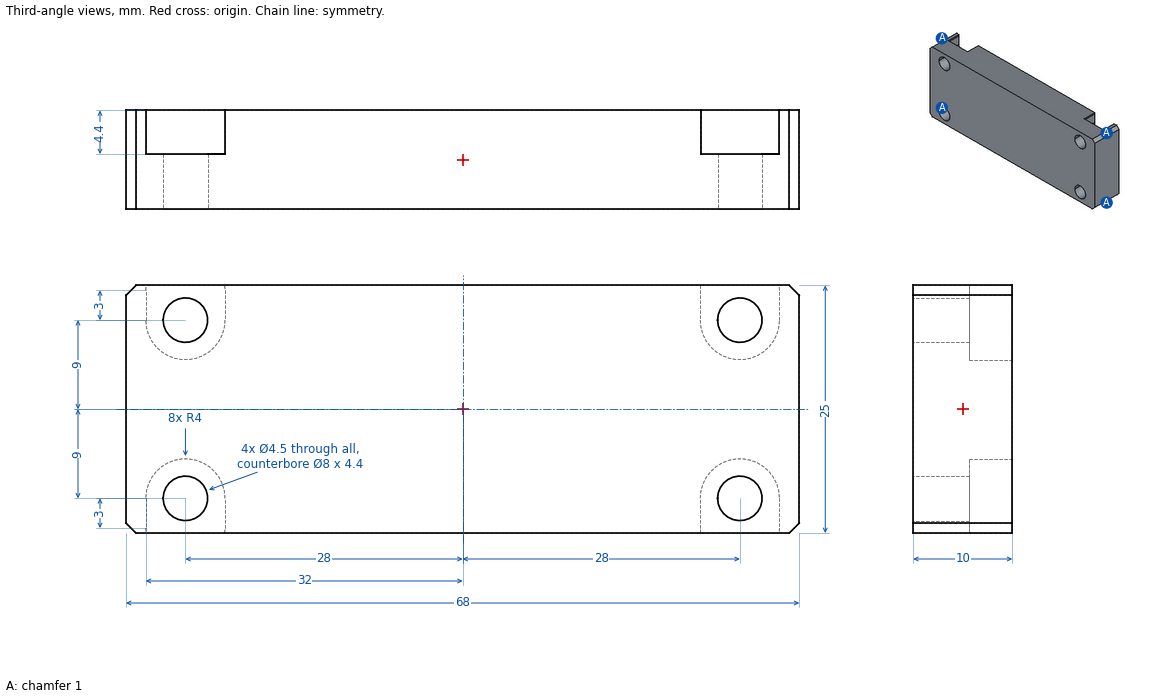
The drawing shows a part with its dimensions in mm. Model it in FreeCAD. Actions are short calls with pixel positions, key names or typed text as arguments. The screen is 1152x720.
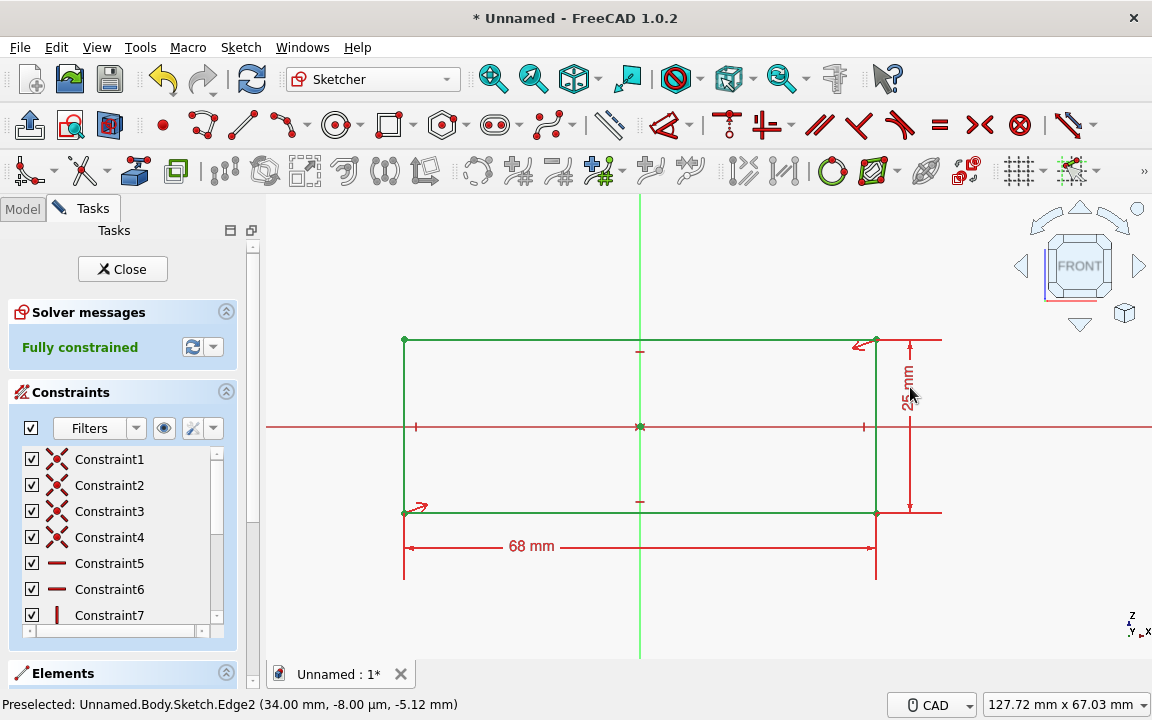
click(123, 269)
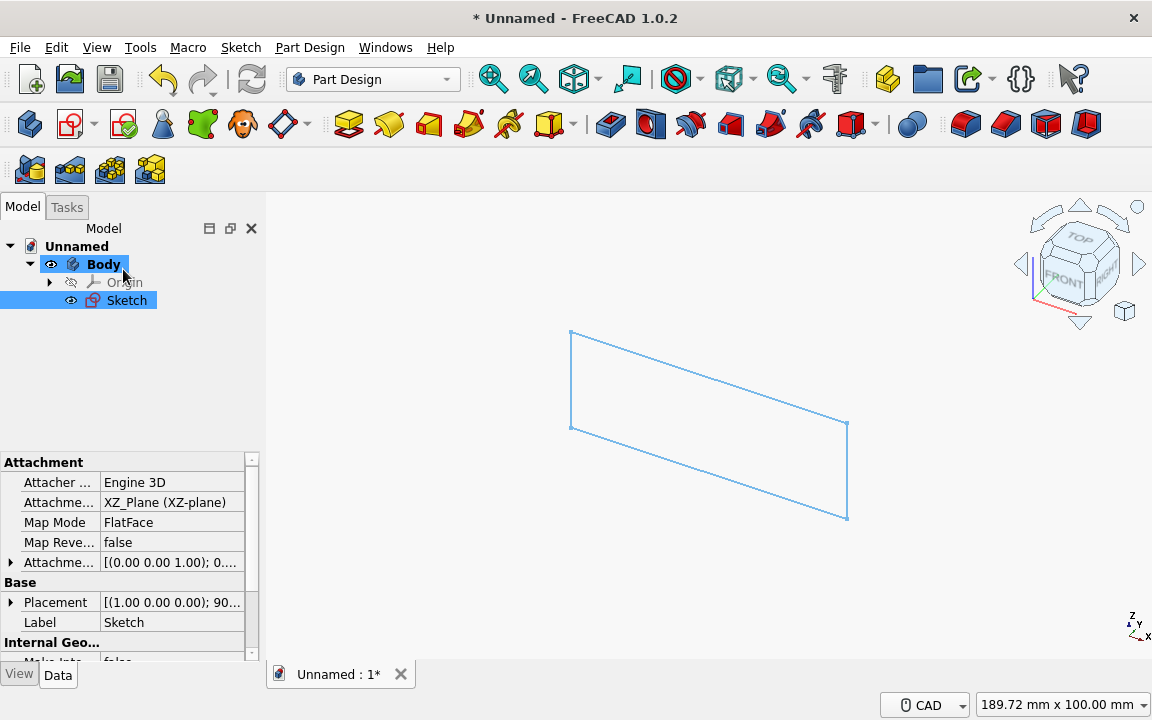
click(350, 124)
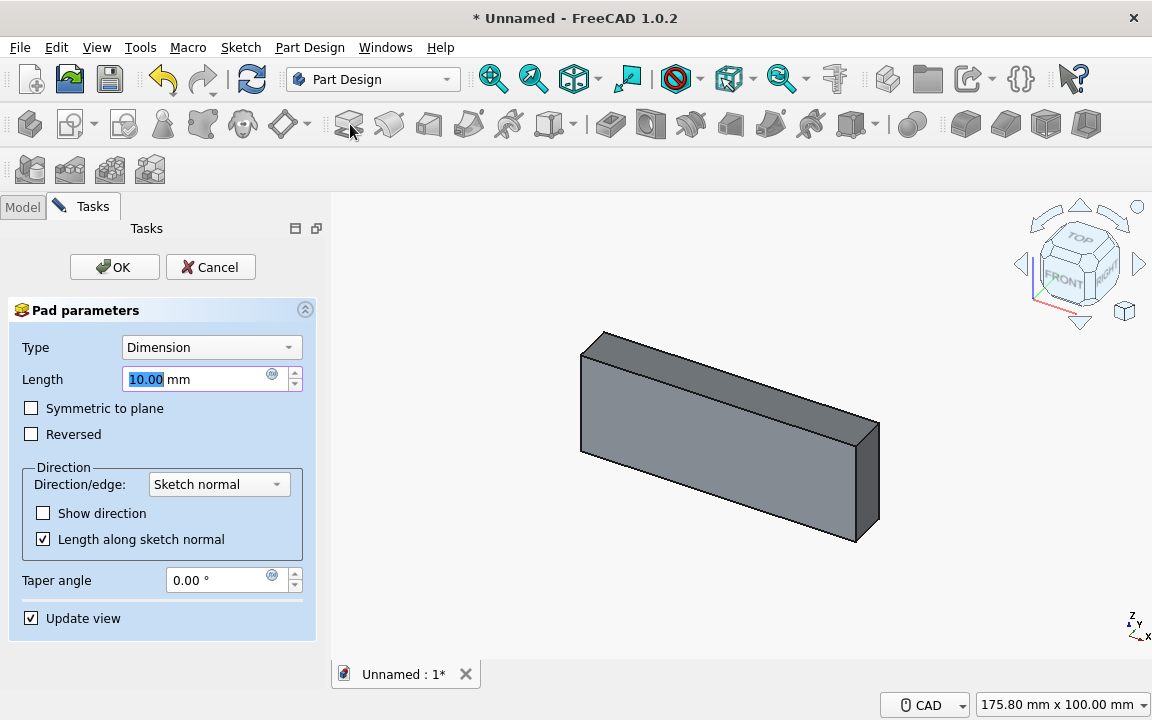
text(10)
key(Tab)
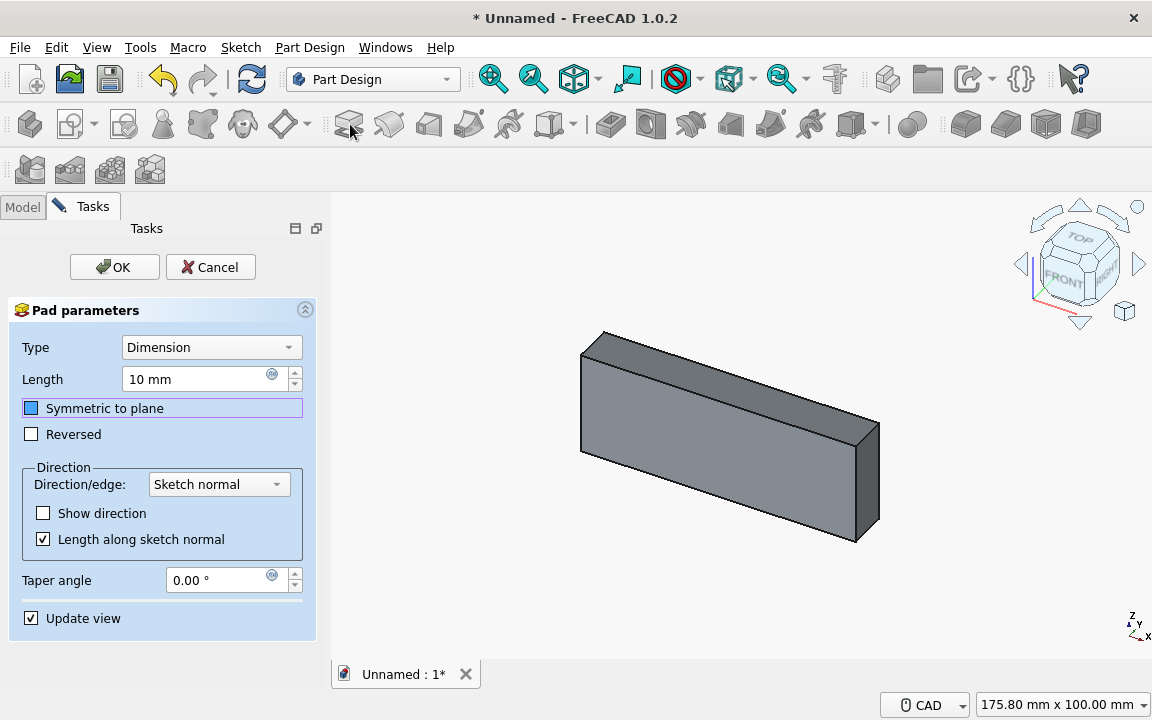
click(30, 408)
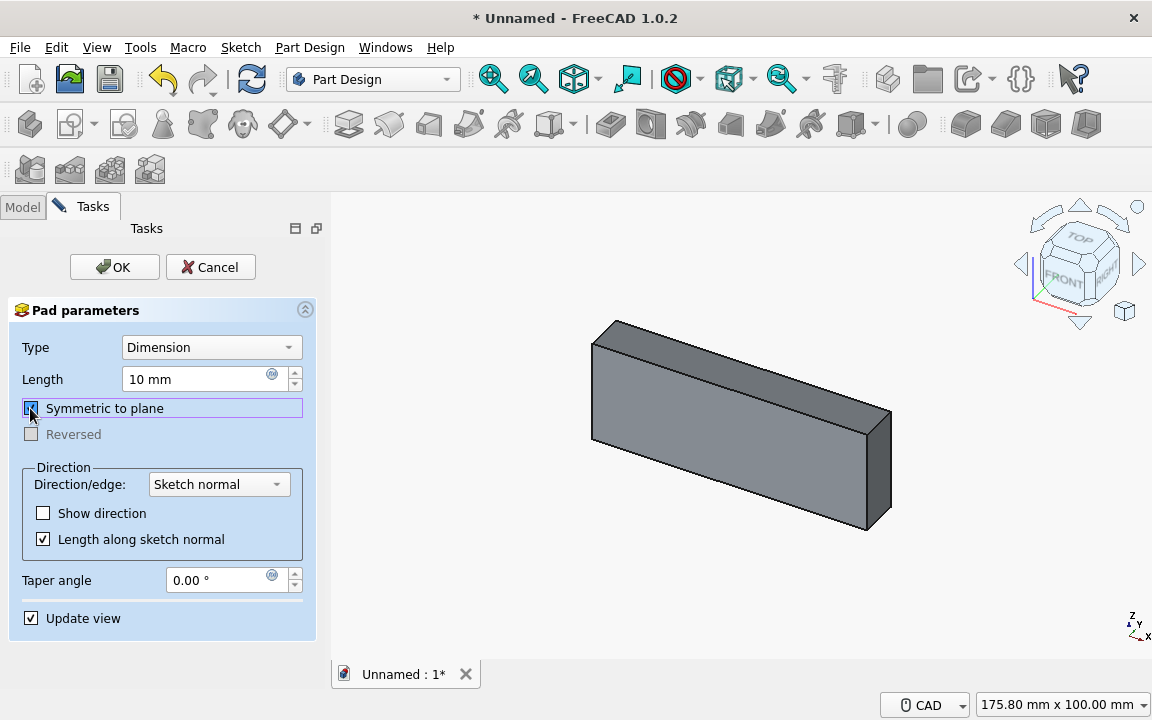
click(115, 267)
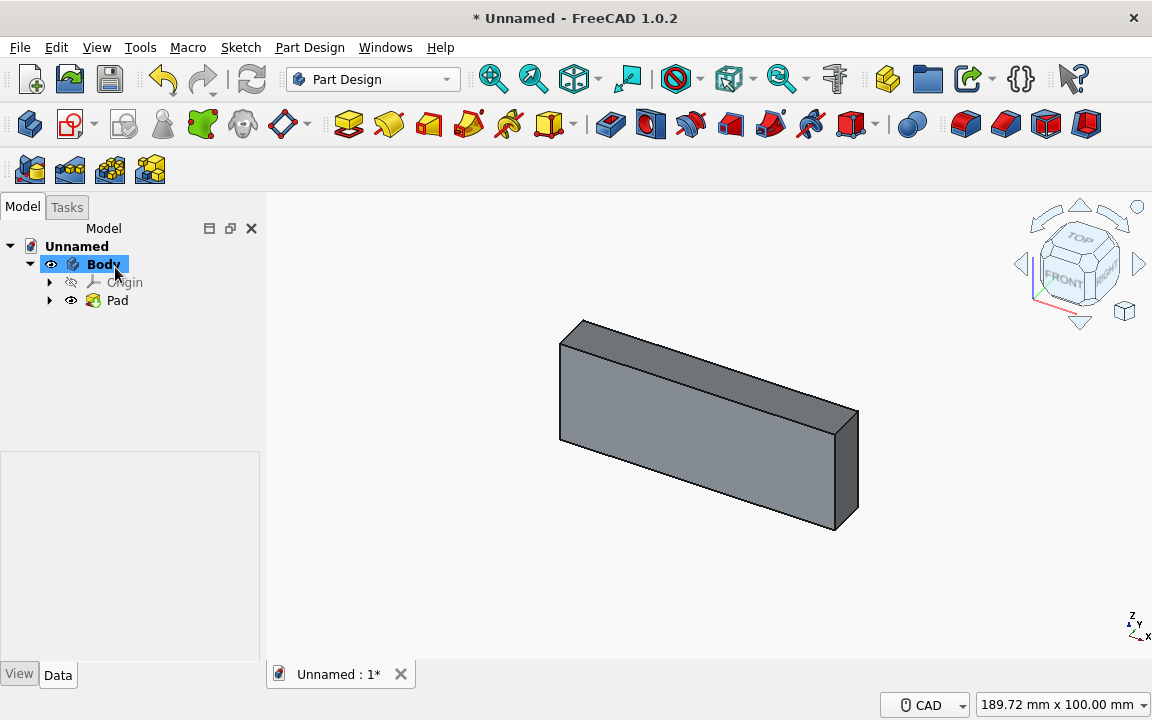
click(494, 80)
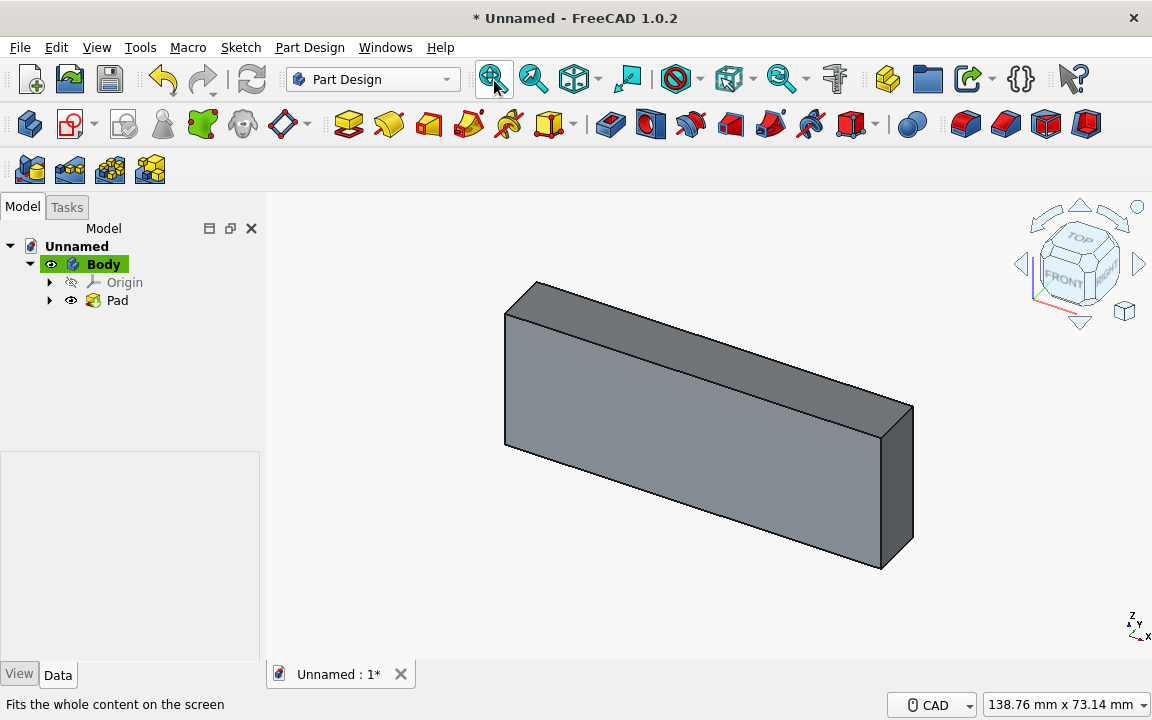
key(4)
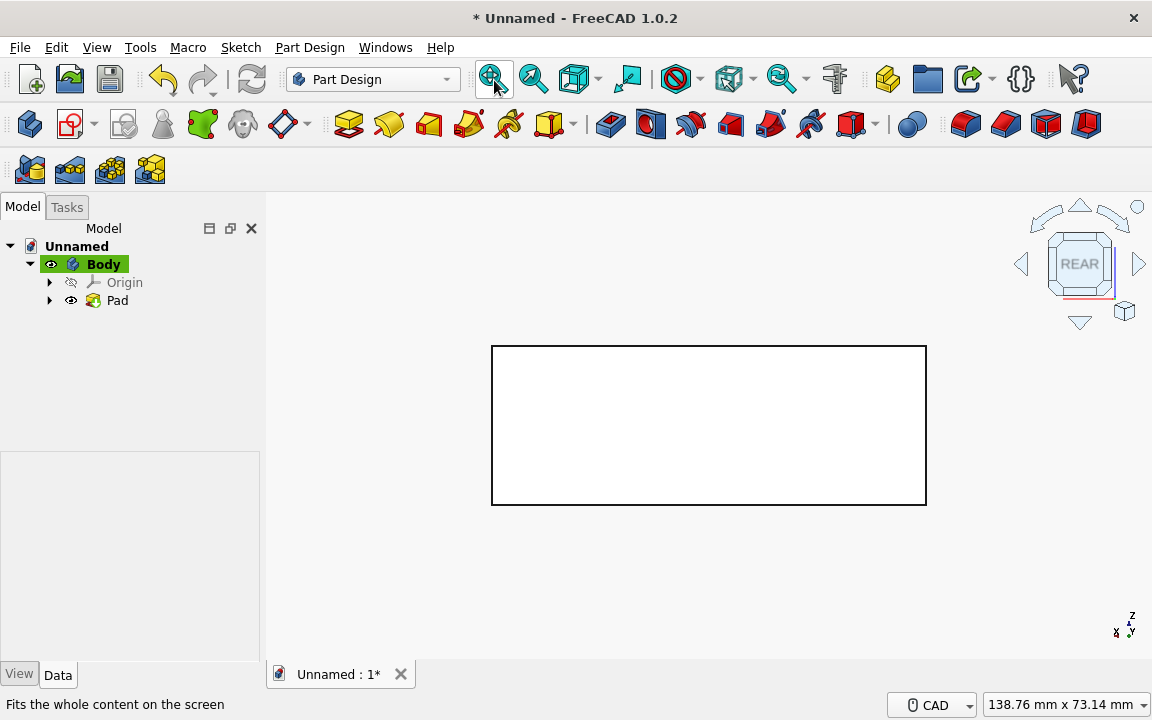
click(585, 424)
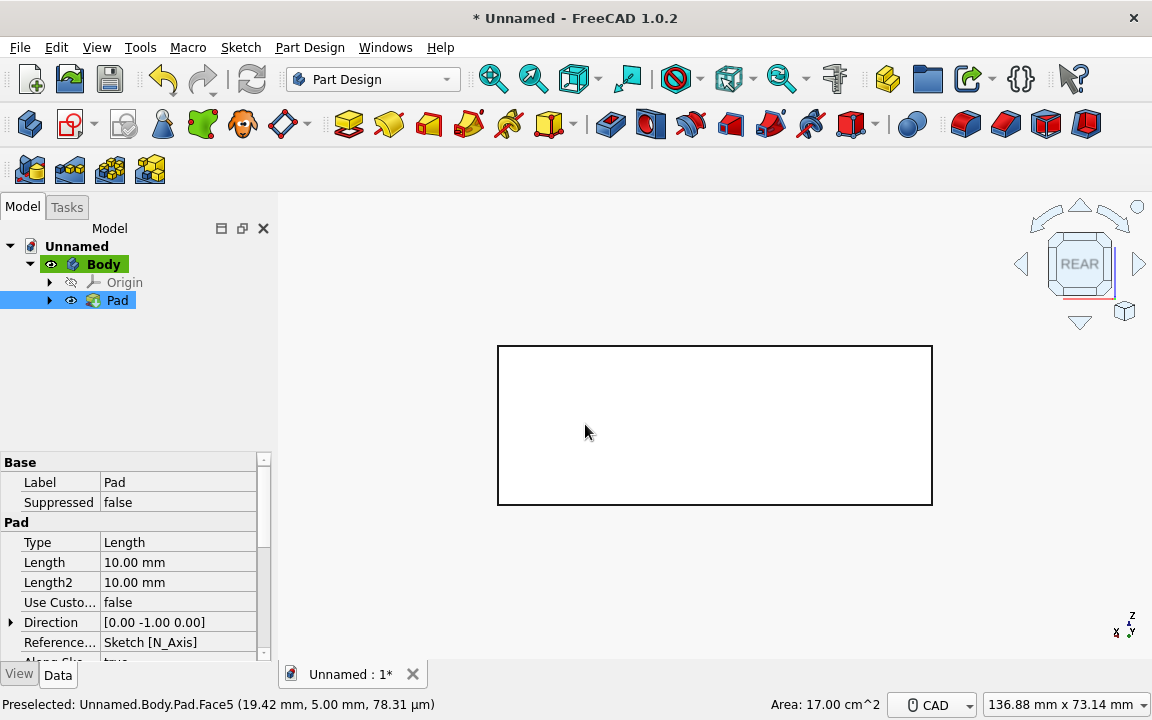
click(70, 124)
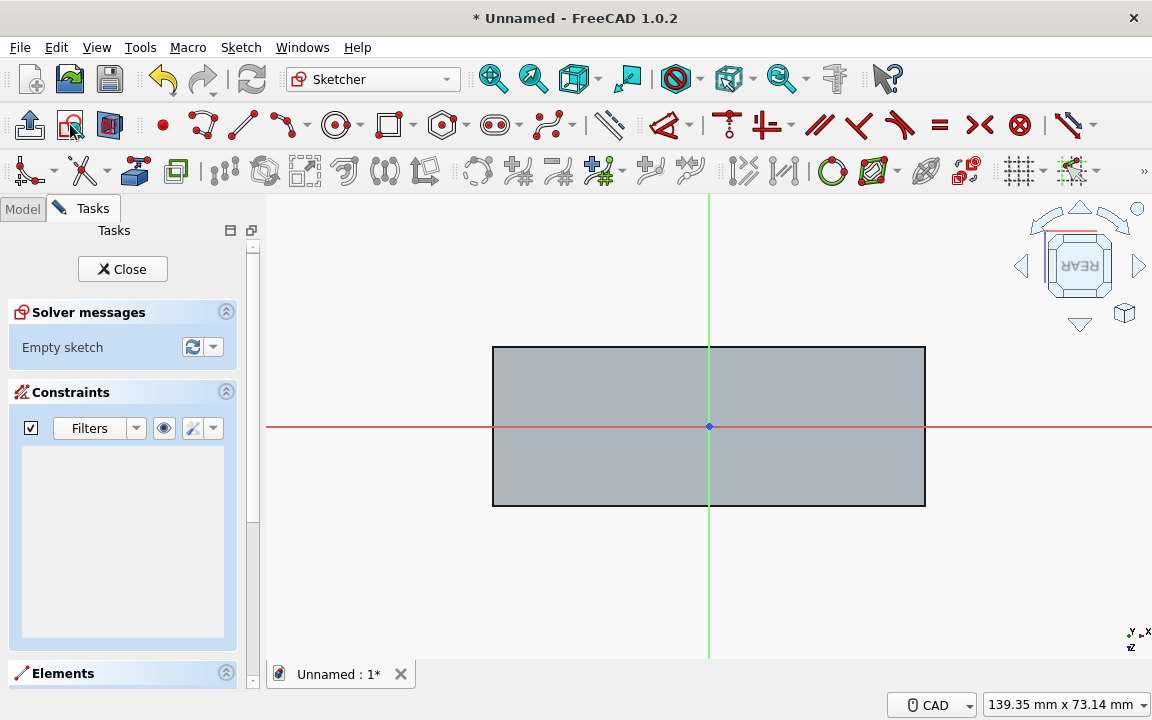
click(336, 126)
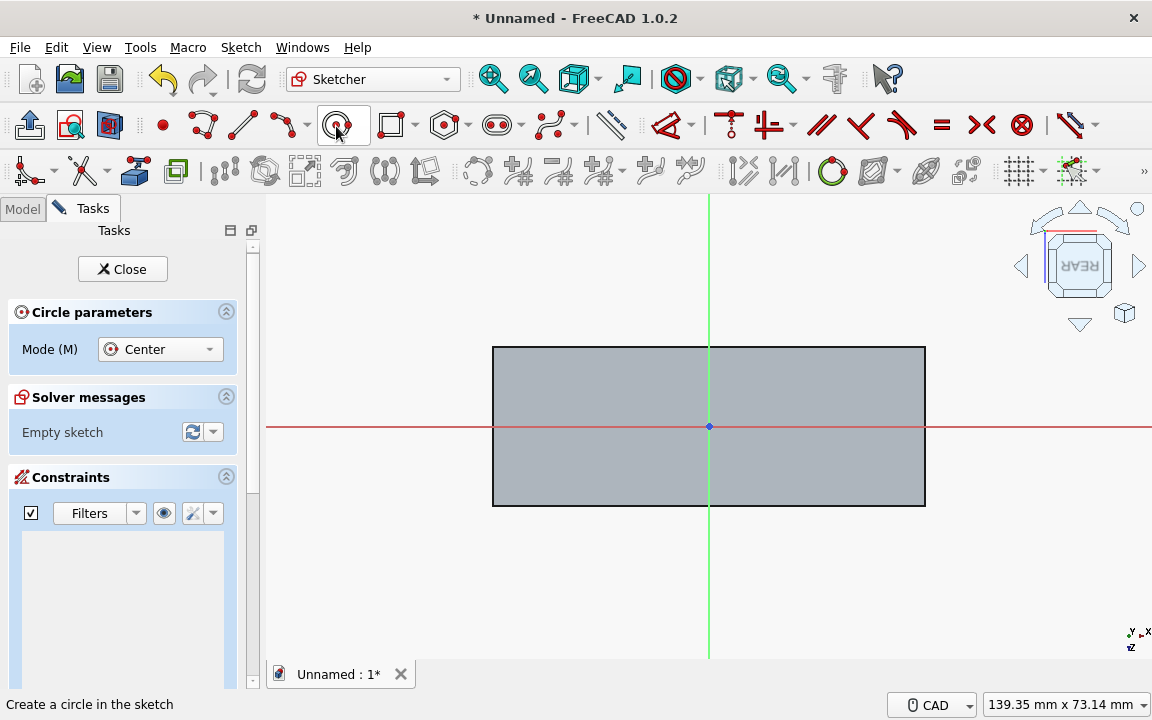
scroll(531, 369, up, 3)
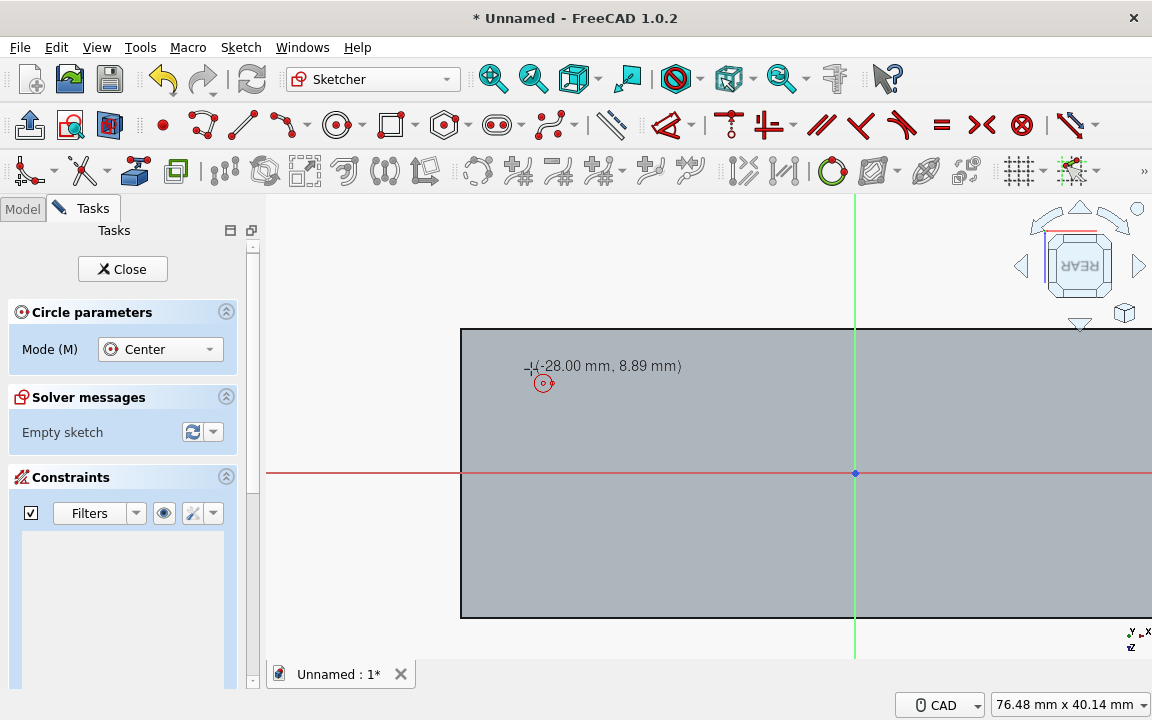
click(531, 369)
click(549, 351)